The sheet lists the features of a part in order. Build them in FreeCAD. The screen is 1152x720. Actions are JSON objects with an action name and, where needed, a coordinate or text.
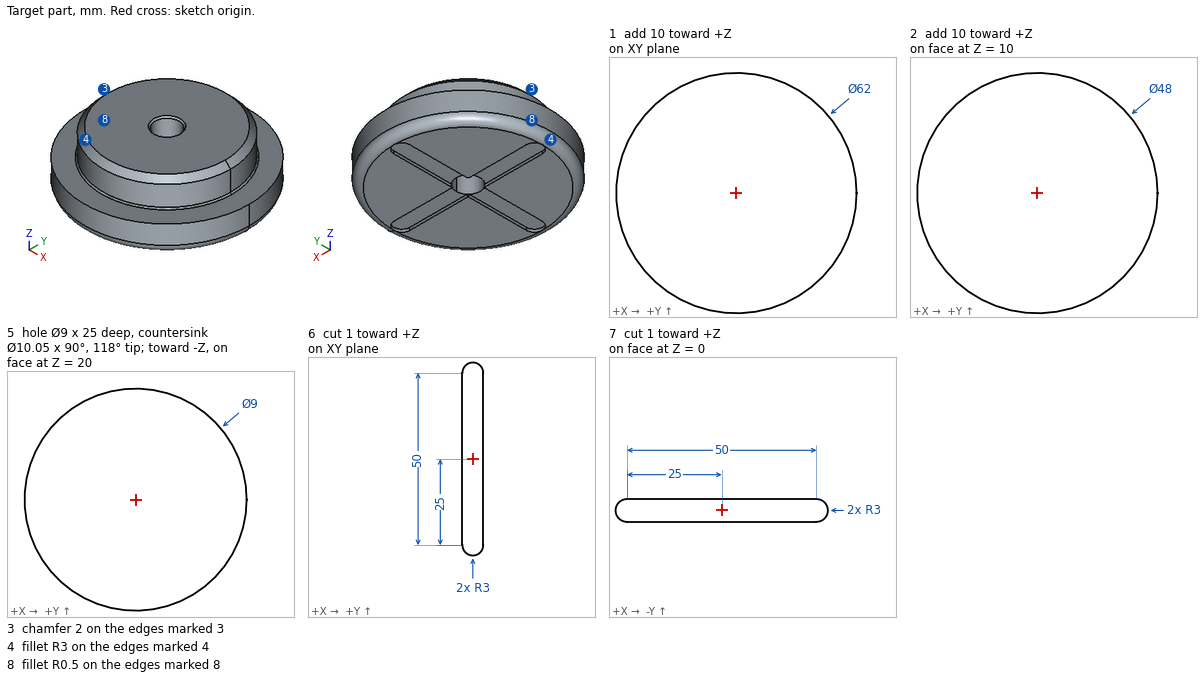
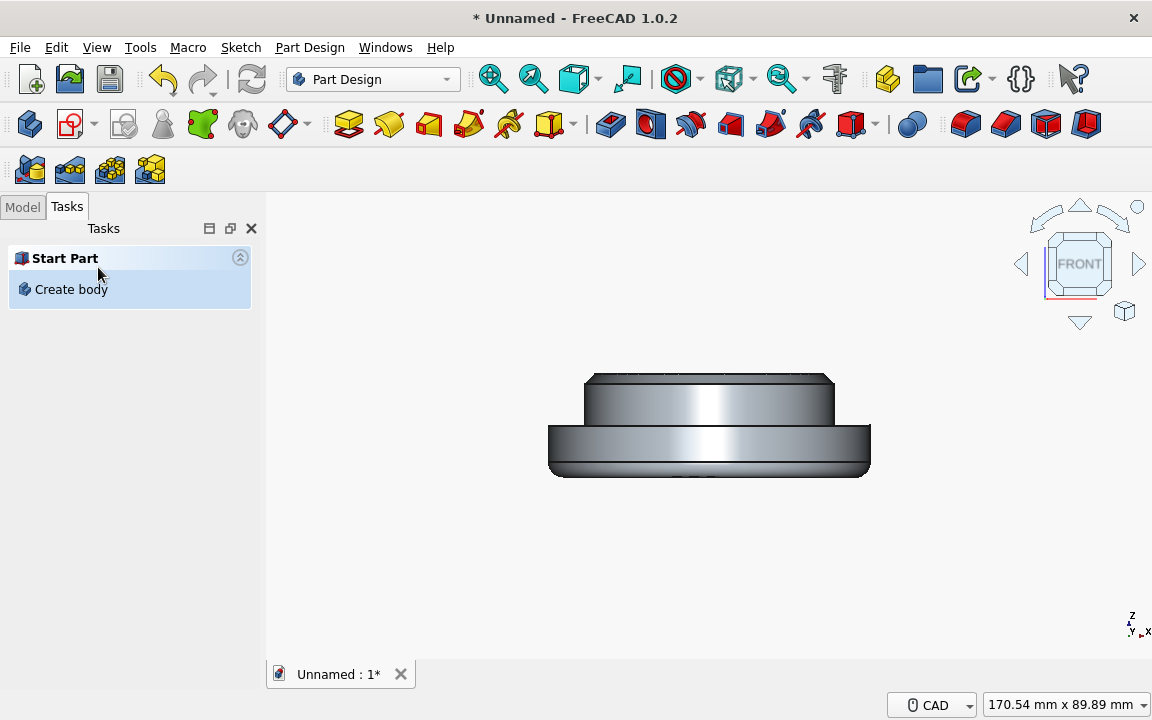
{"action": "key", "text": "v f"}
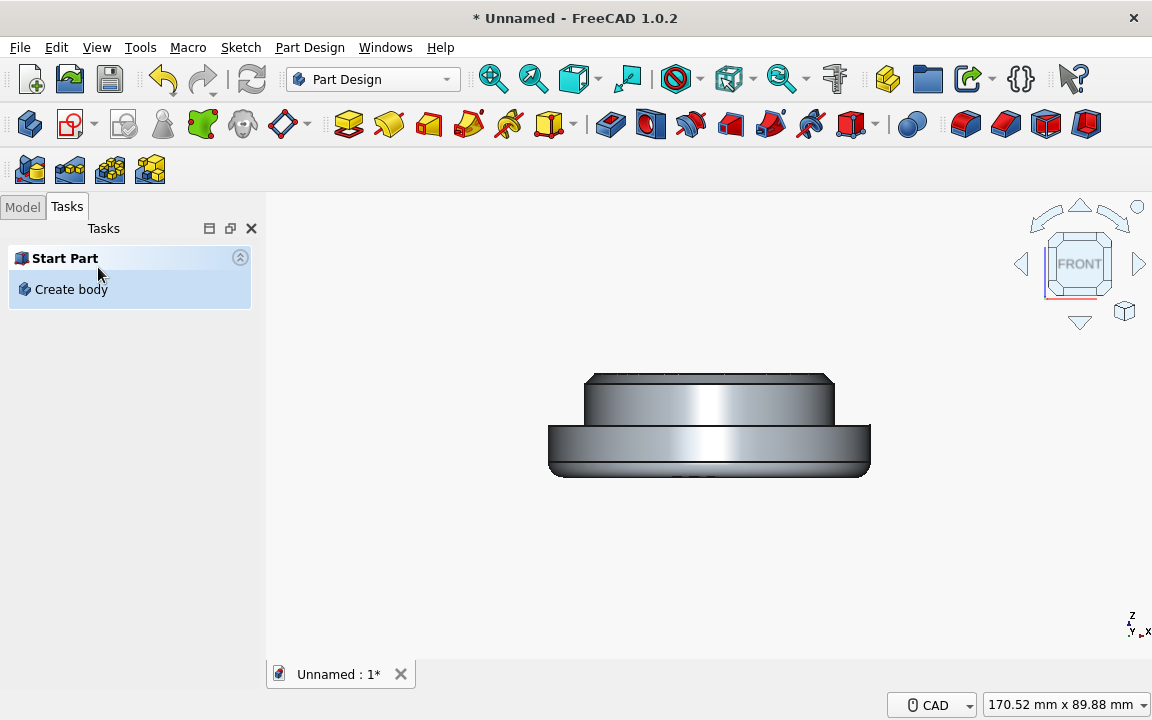
{"action": "key", "text": "0"}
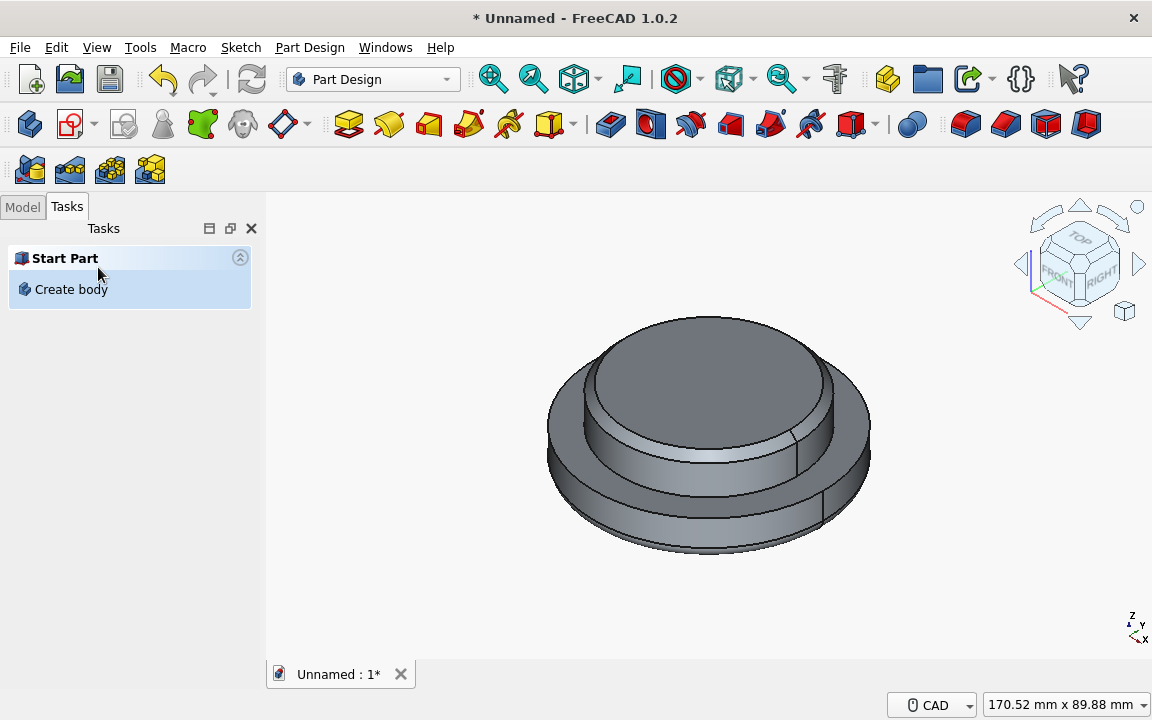
{"action": "left_click", "coordinate": [709, 382]}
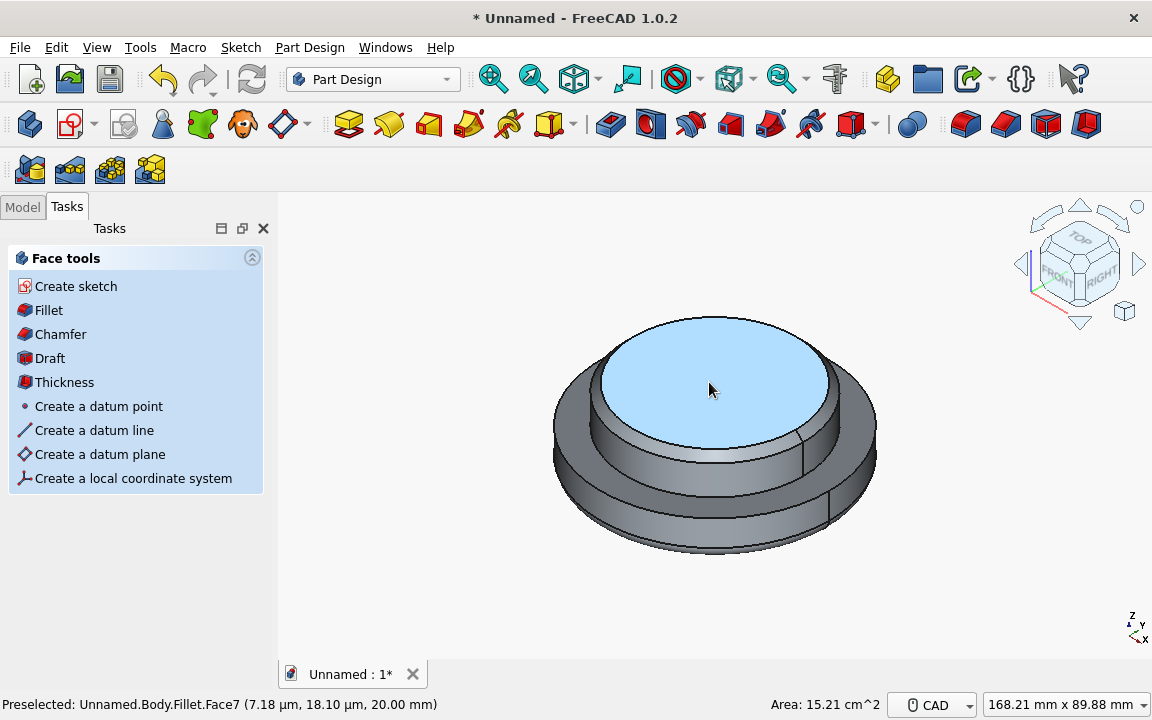
{"action": "left_click", "coordinate": [70, 124]}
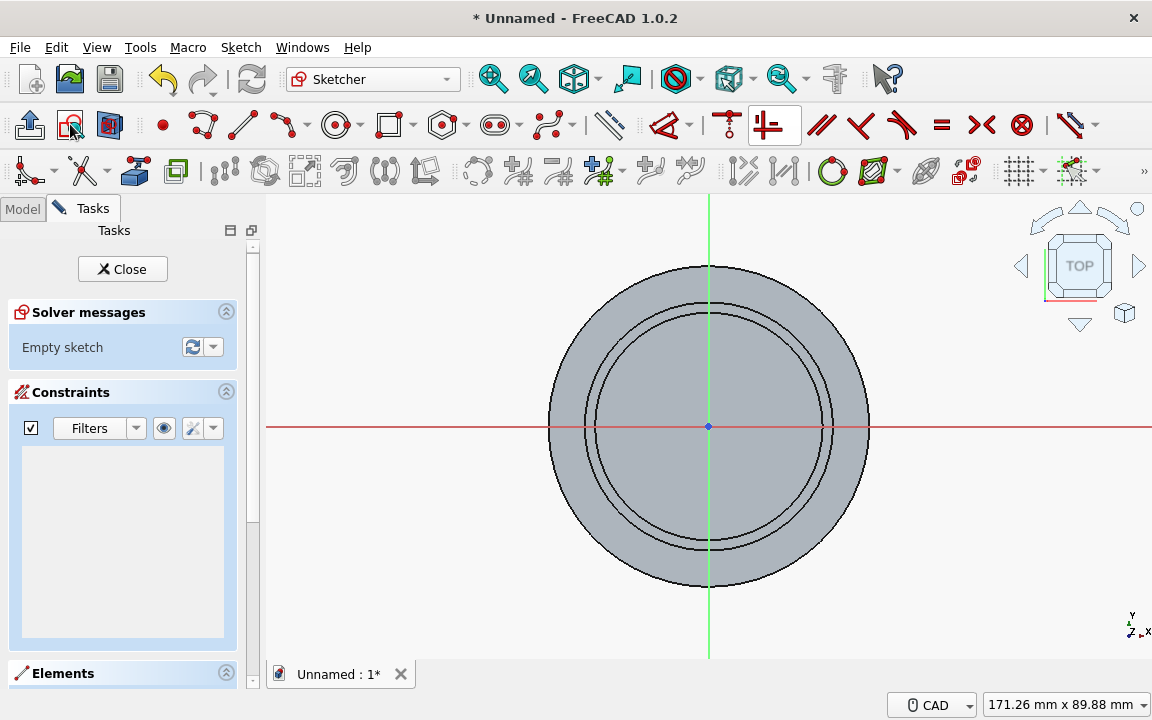
{"action": "scroll", "coordinate": [722, 427], "scroll_direction": "up", "scroll_amount": 9}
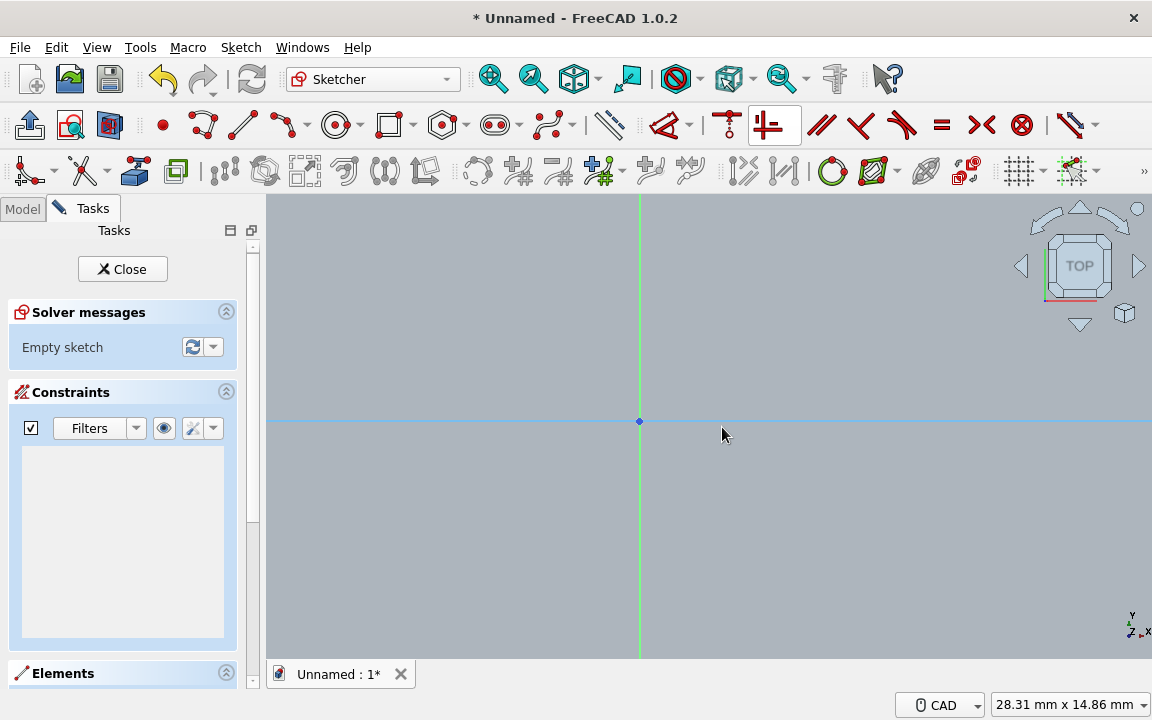
{"action": "left_click", "coordinate": [336, 126]}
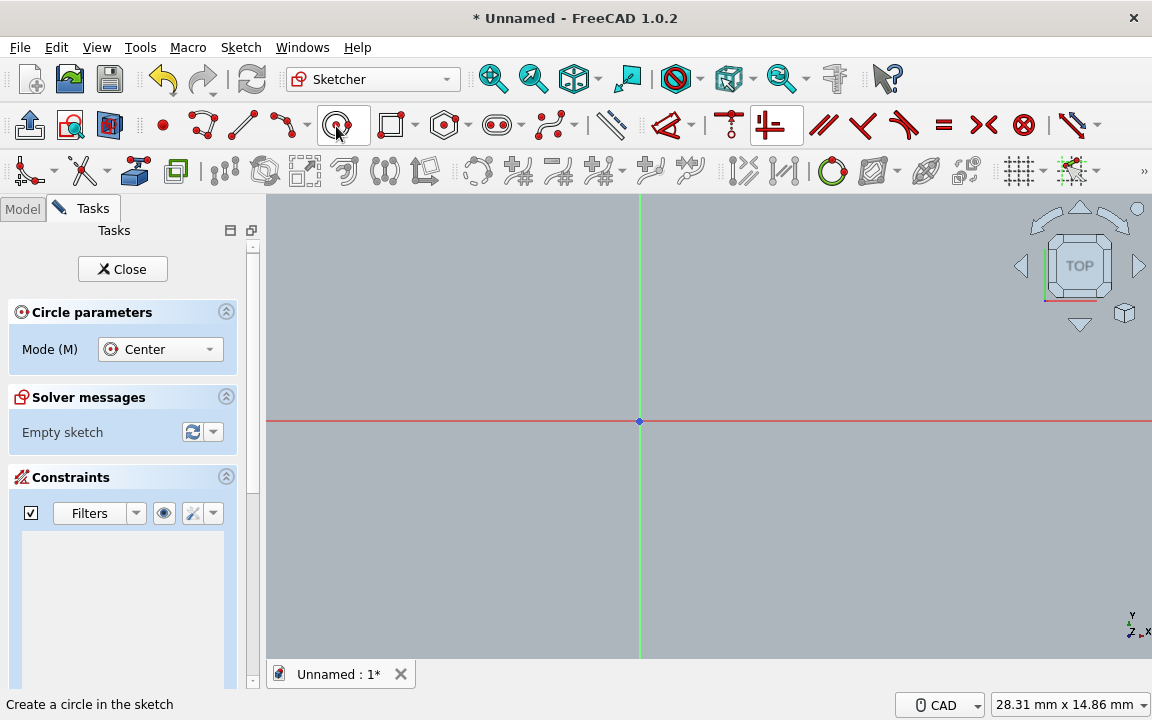
{"action": "left_click", "coordinate": [640, 421]}
{"action": "left_click", "coordinate": [740, 322]}
{"action": "key", "text": "Escape"}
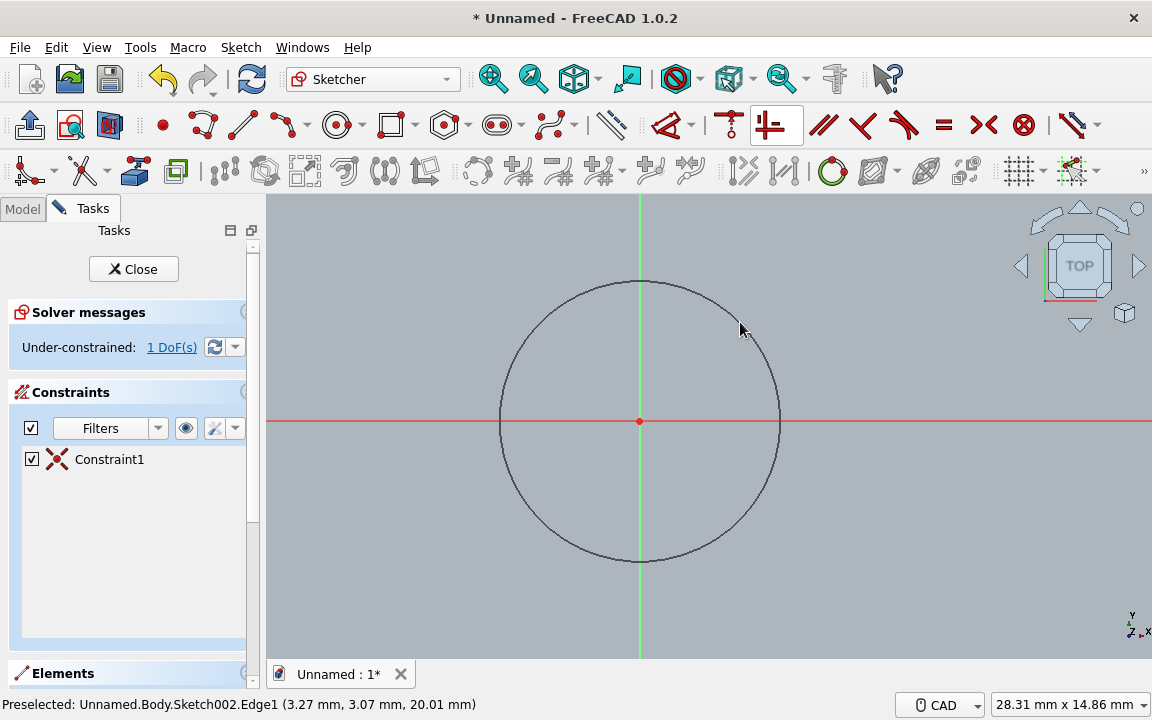
{"action": "left_click", "coordinate": [666, 126]}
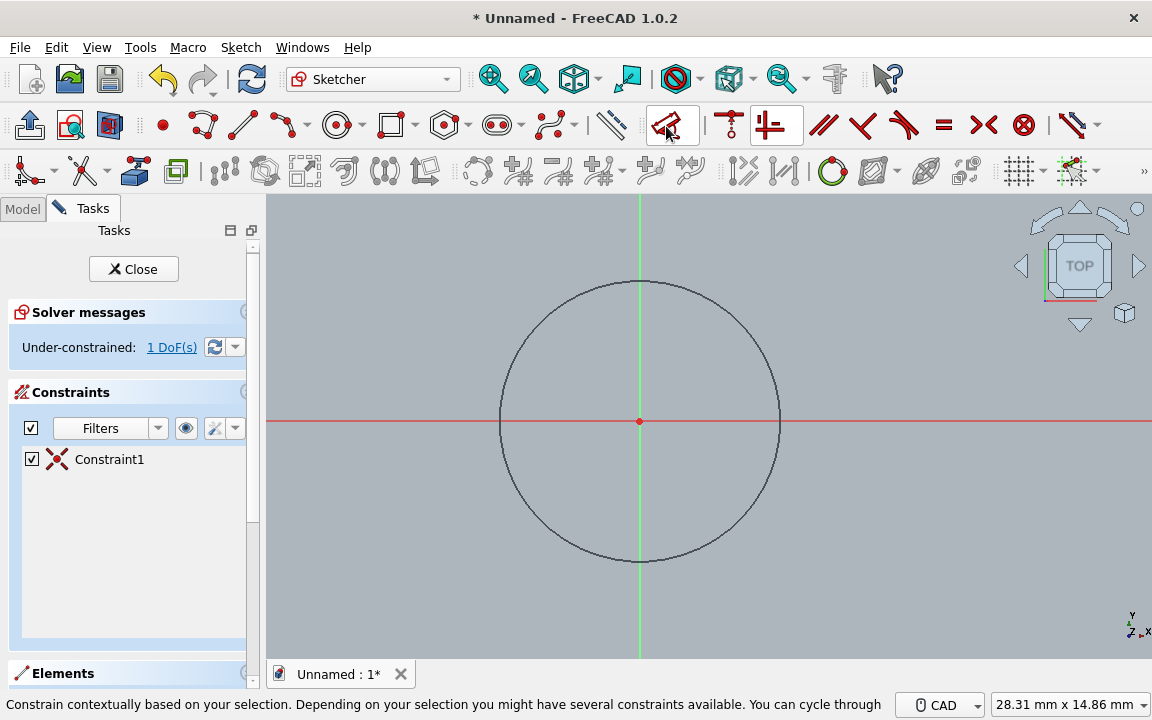
{"action": "left_click", "coordinate": [739, 322]}
{"action": "left_click", "coordinate": [762, 299]}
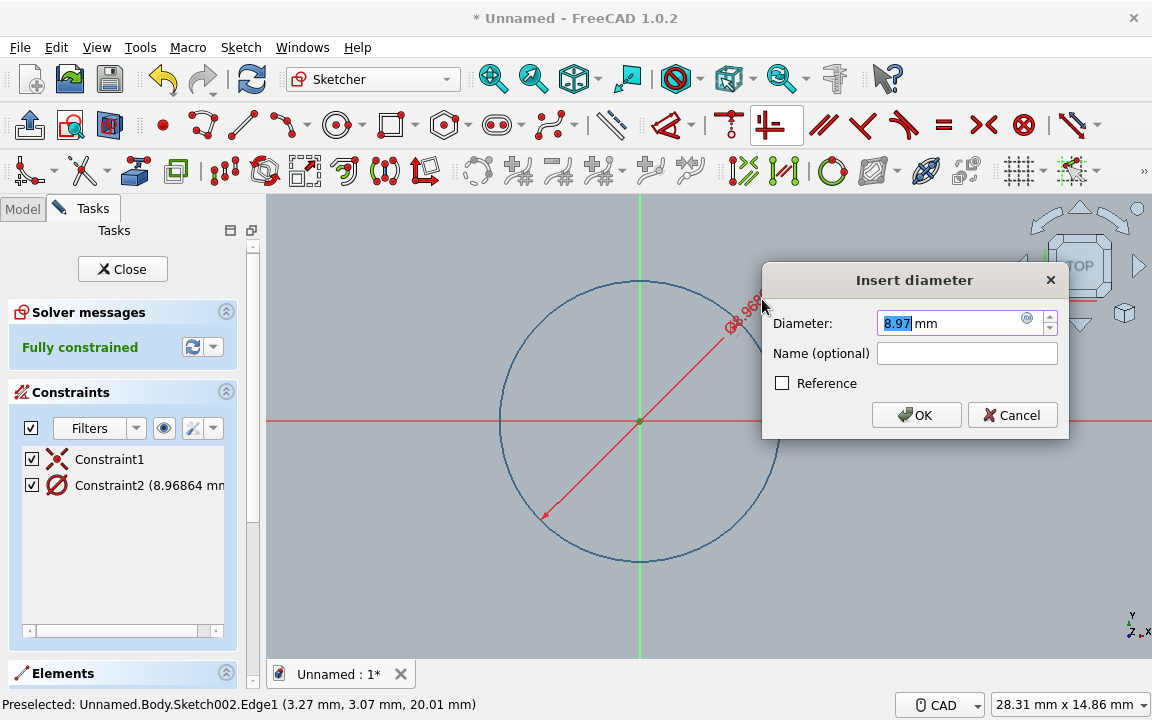
{"action": "type", "text": "9"}
{"action": "key", "text": "Return"}
{"action": "key", "text": "Escape"}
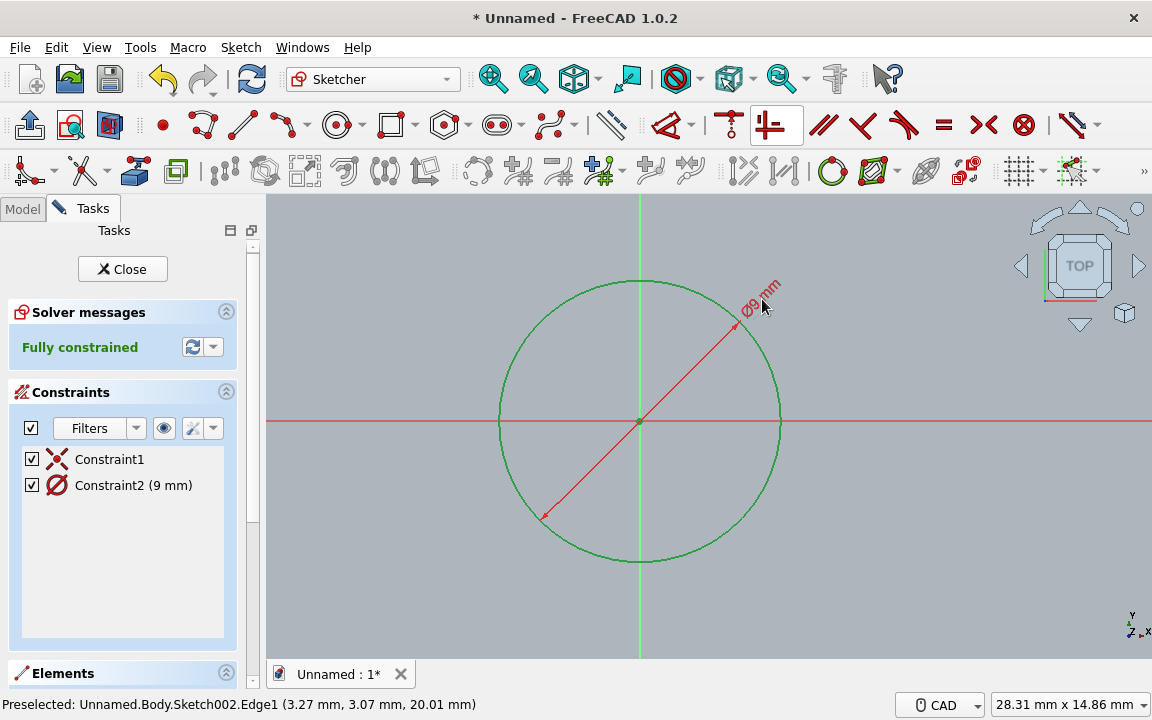
{"action": "left_click", "coordinate": [123, 269]}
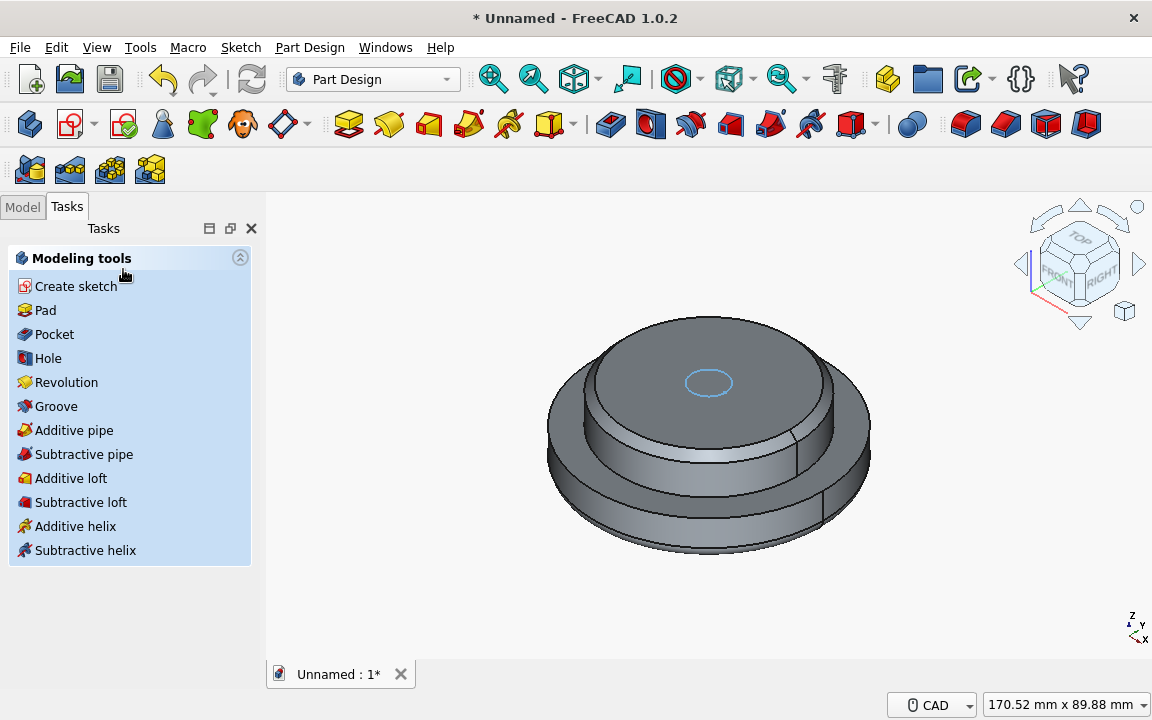
{"action": "left_click", "coordinate": [652, 124]}